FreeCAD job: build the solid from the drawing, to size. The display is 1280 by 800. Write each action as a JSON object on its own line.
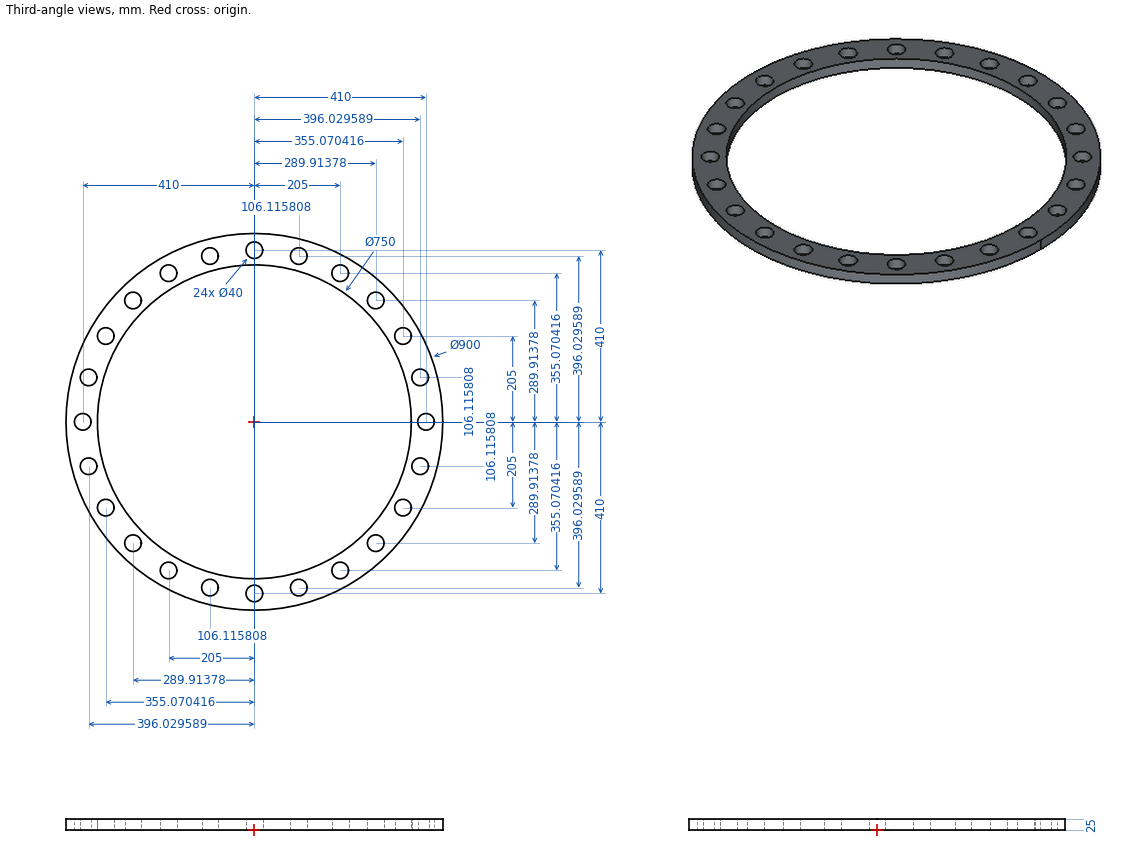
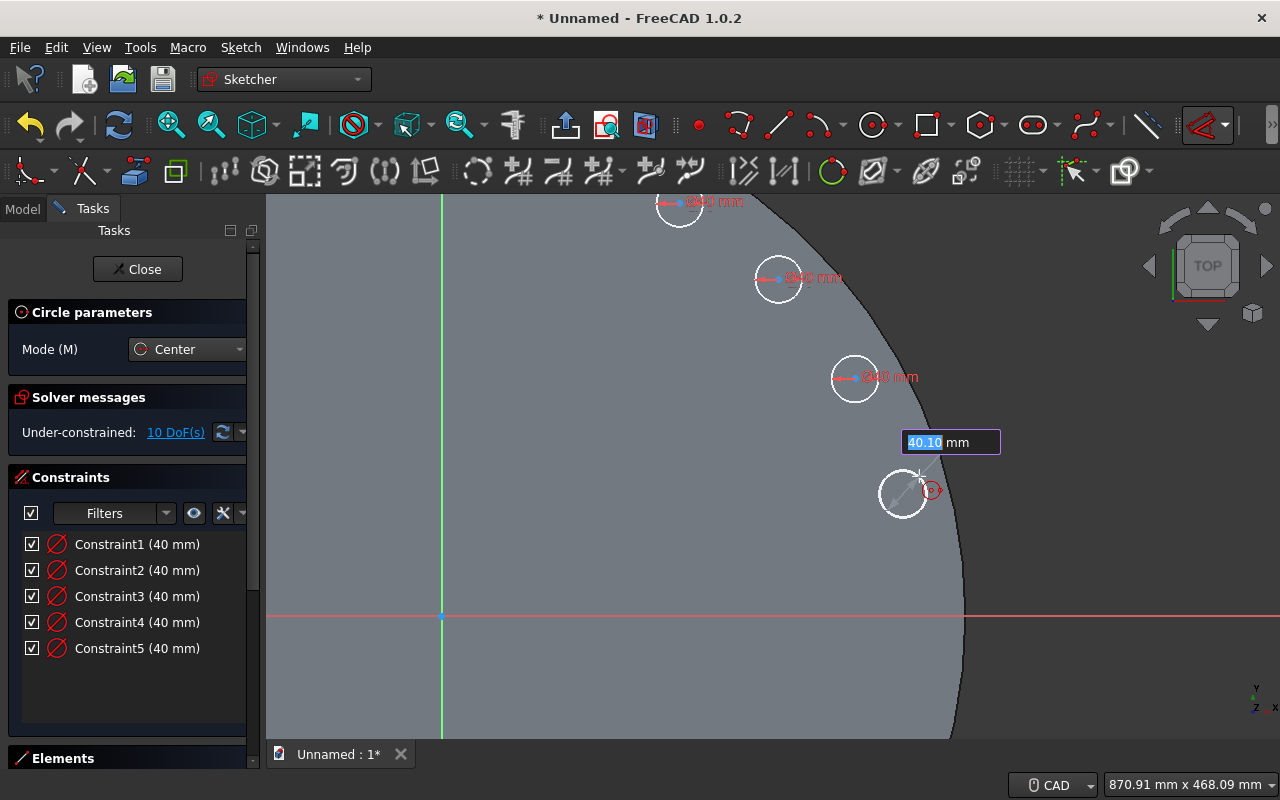
{"action": "type", "text": "40"}
{"action": "key", "text": "Return"}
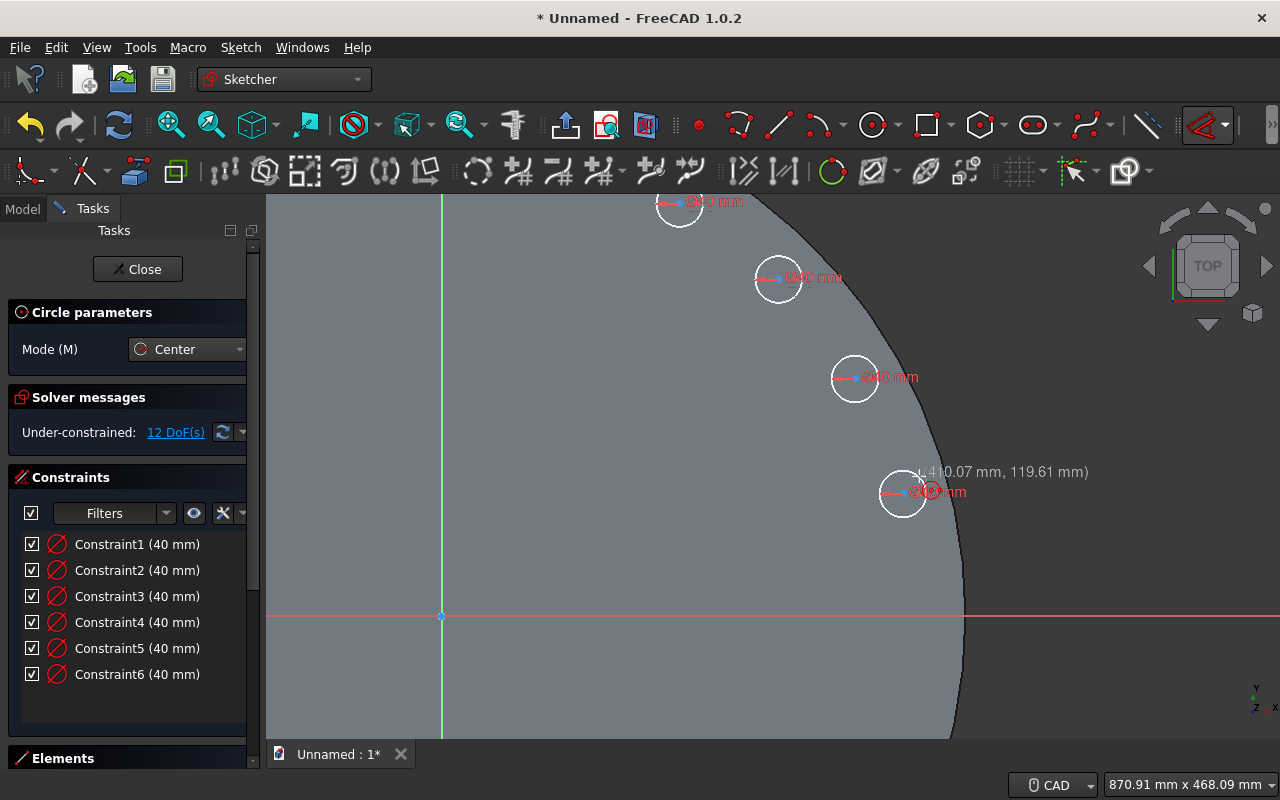
{"action": "left_click", "coordinate": [919, 616]}
{"action": "mouse_move", "coordinate": [935, 600]}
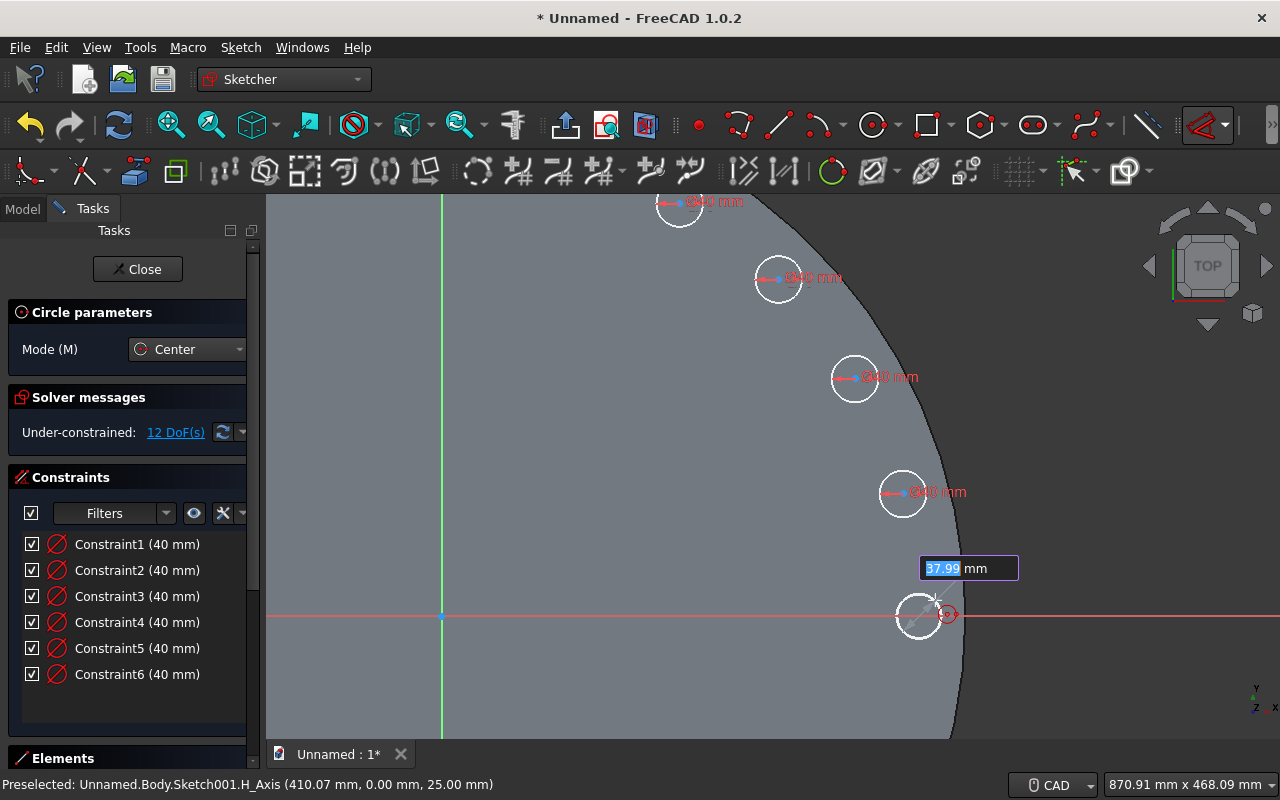
{"action": "type", "text": "40"}
{"action": "key", "text": "Return"}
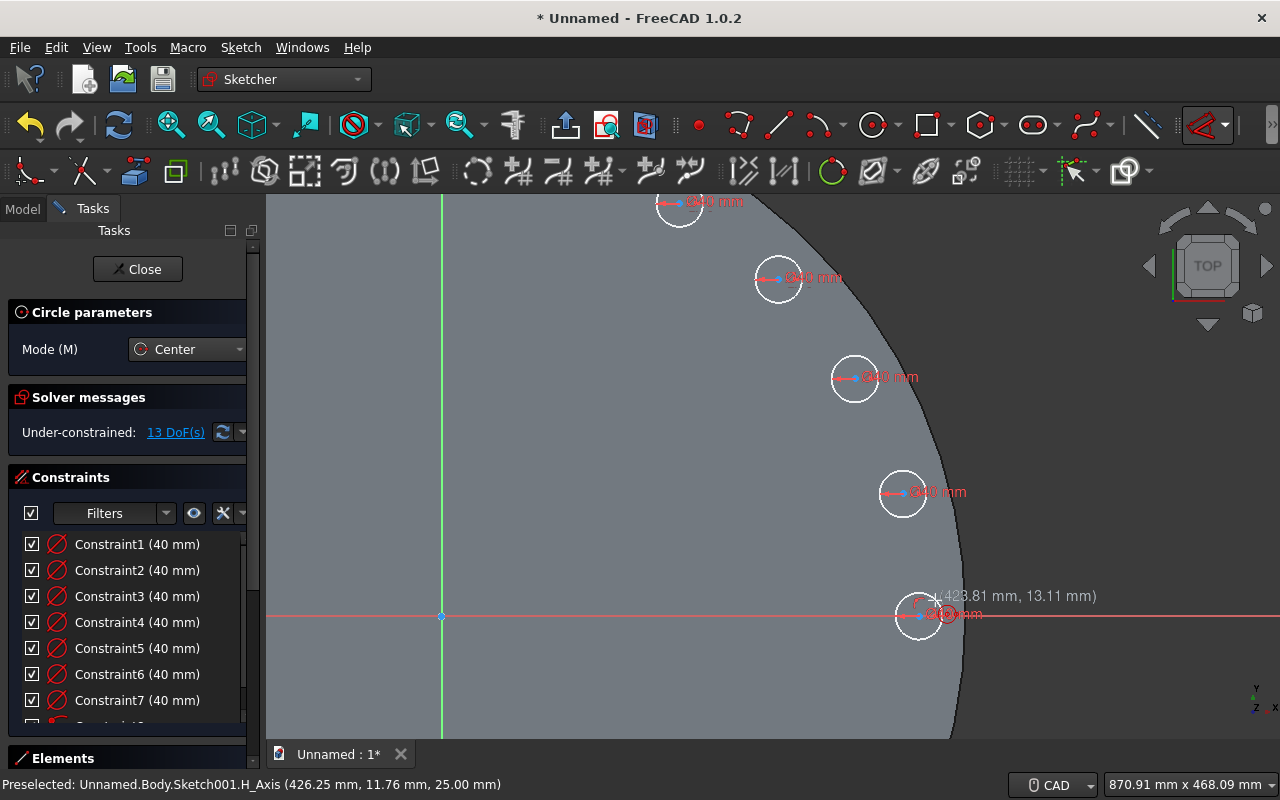
{"action": "scroll", "coordinate": [858, 379], "scroll_direction": "down", "scroll_amount": 5}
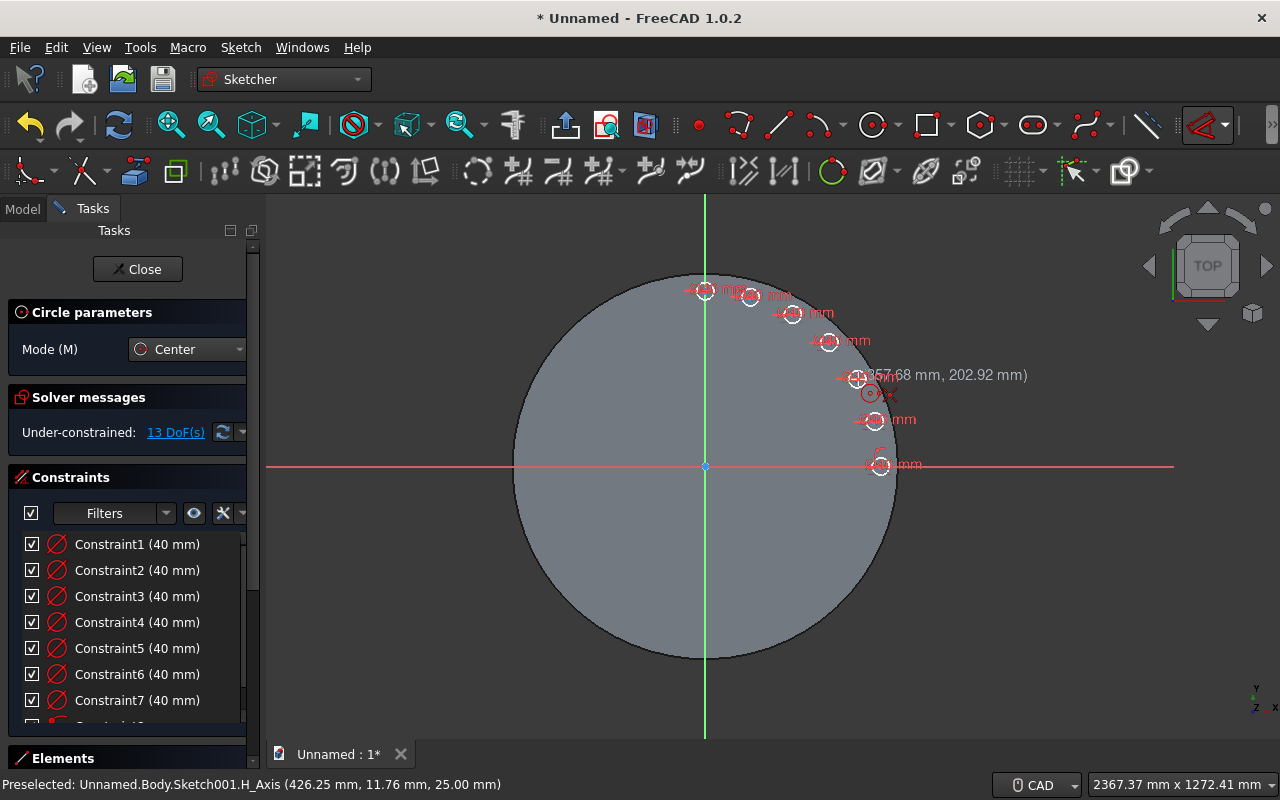
{"action": "scroll", "coordinate": [875, 512], "scroll_direction": "up", "scroll_amount": 5}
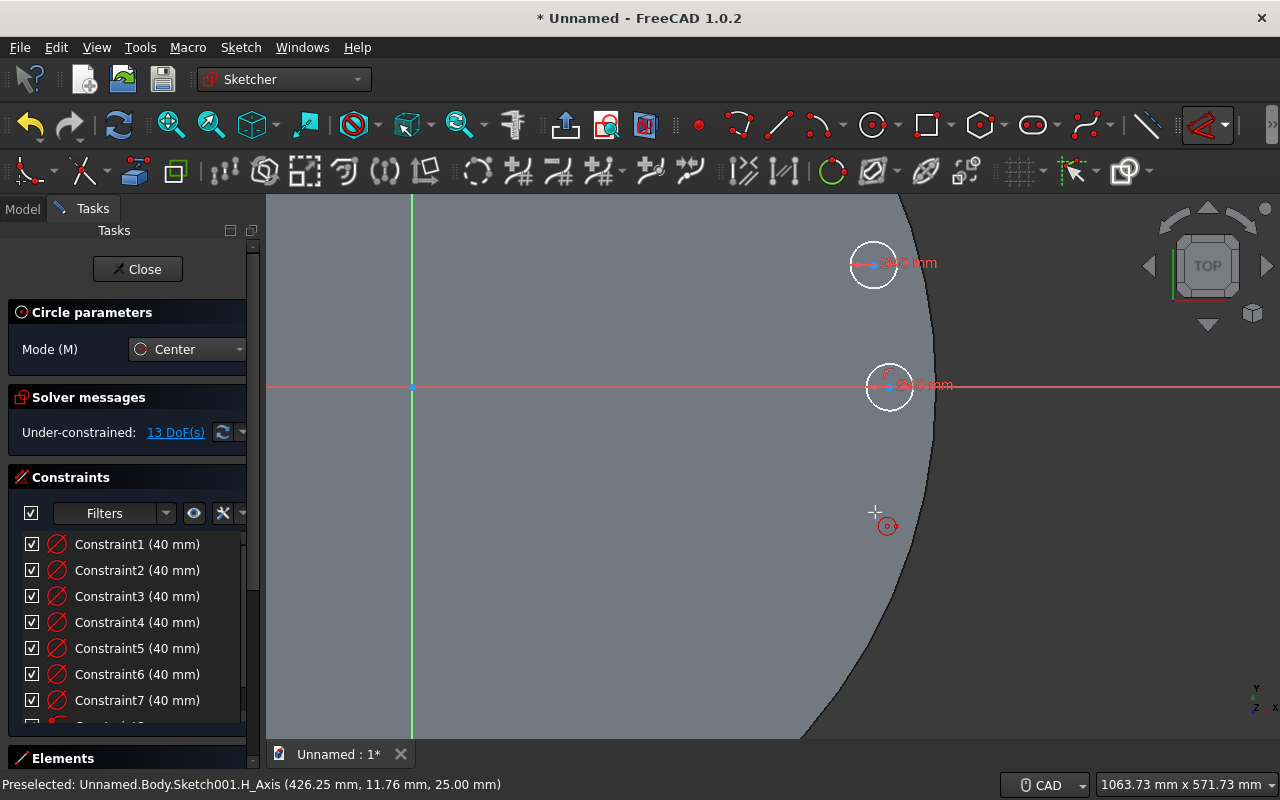
{"action": "left_click", "coordinate": [873, 511]}
{"action": "mouse_move", "coordinate": [890, 494]}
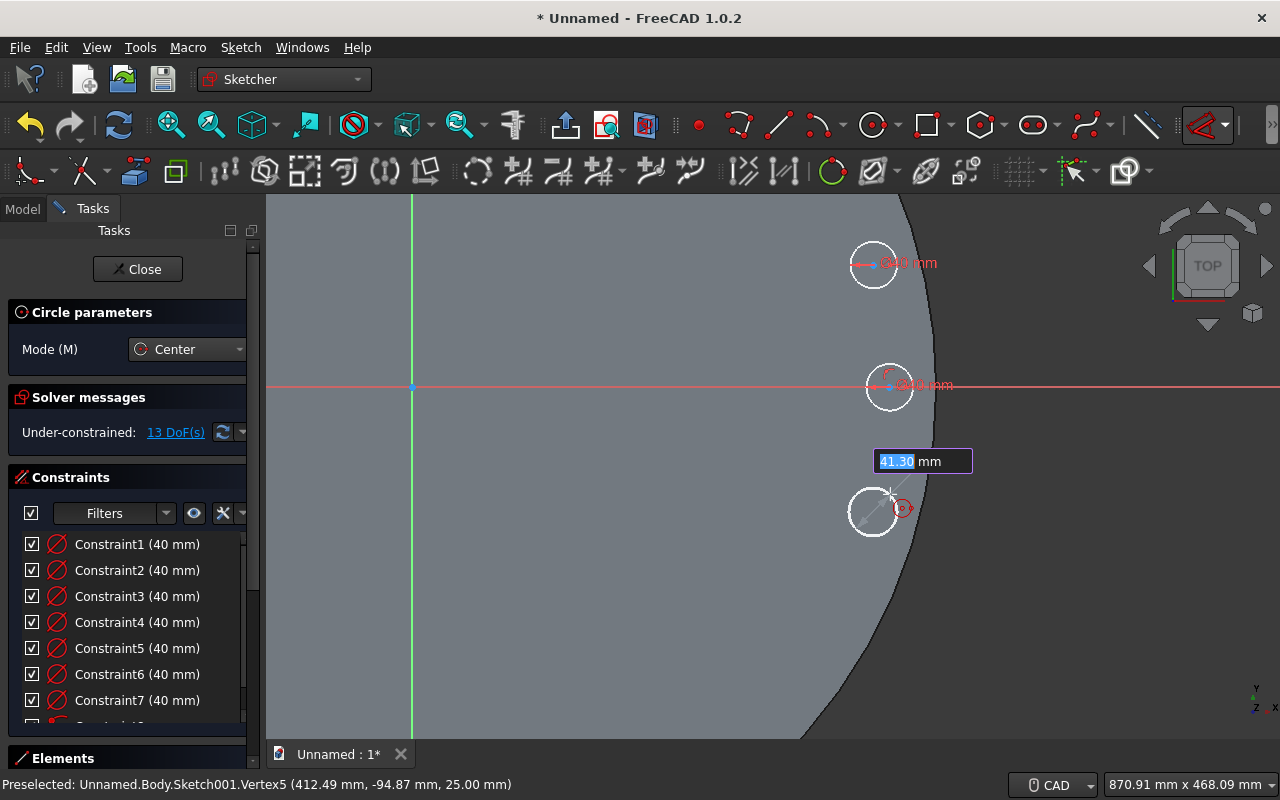
{"action": "type", "text": "40"}
{"action": "key", "text": "Return"}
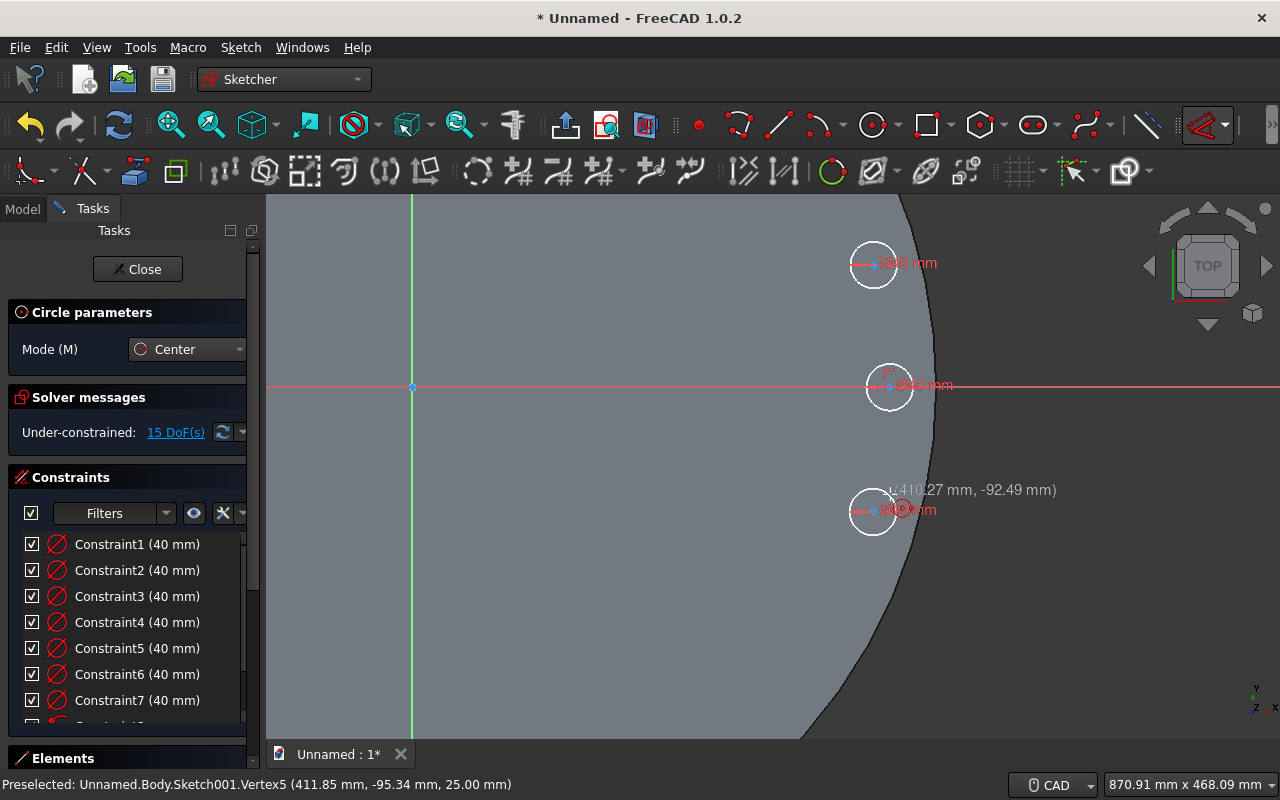
{"action": "left_click", "coordinate": [826, 626]}
{"action": "mouse_move", "coordinate": [842, 610]}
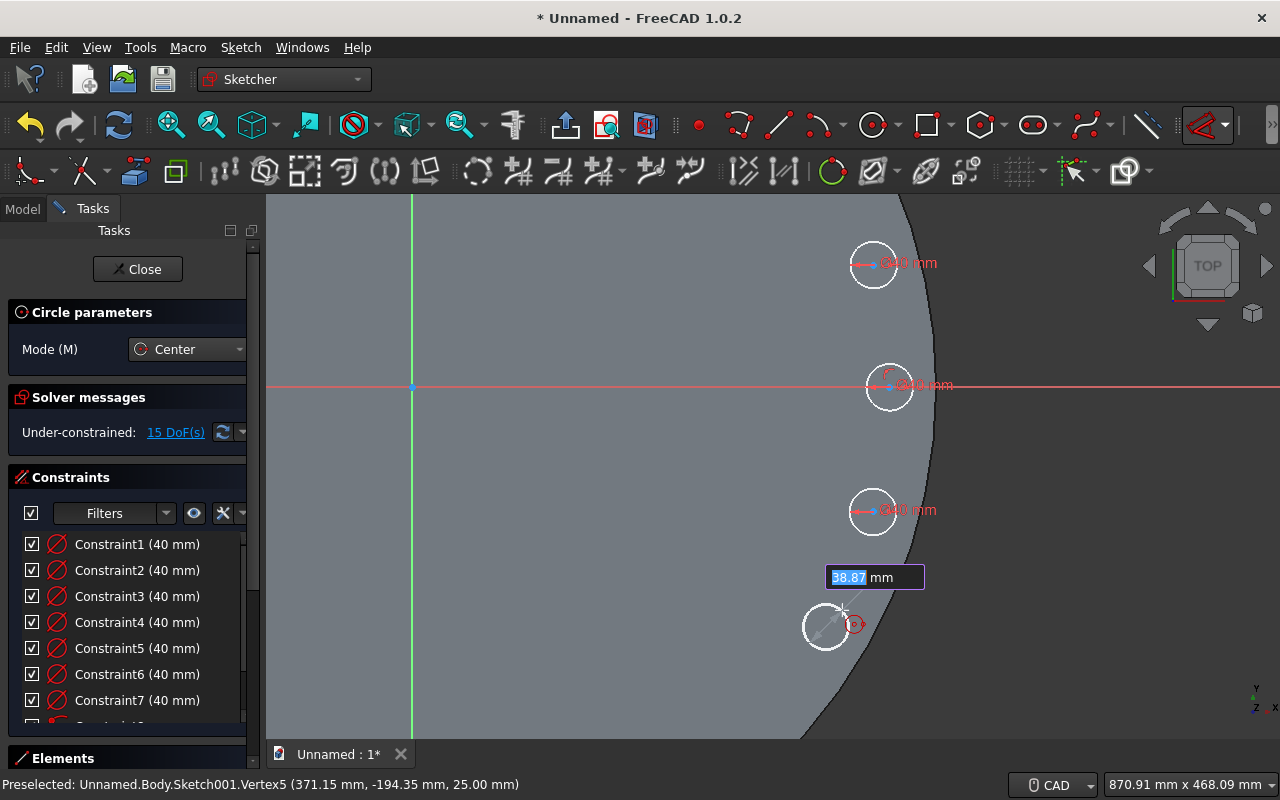
{"action": "type", "text": "40"}
{"action": "key", "text": "Return"}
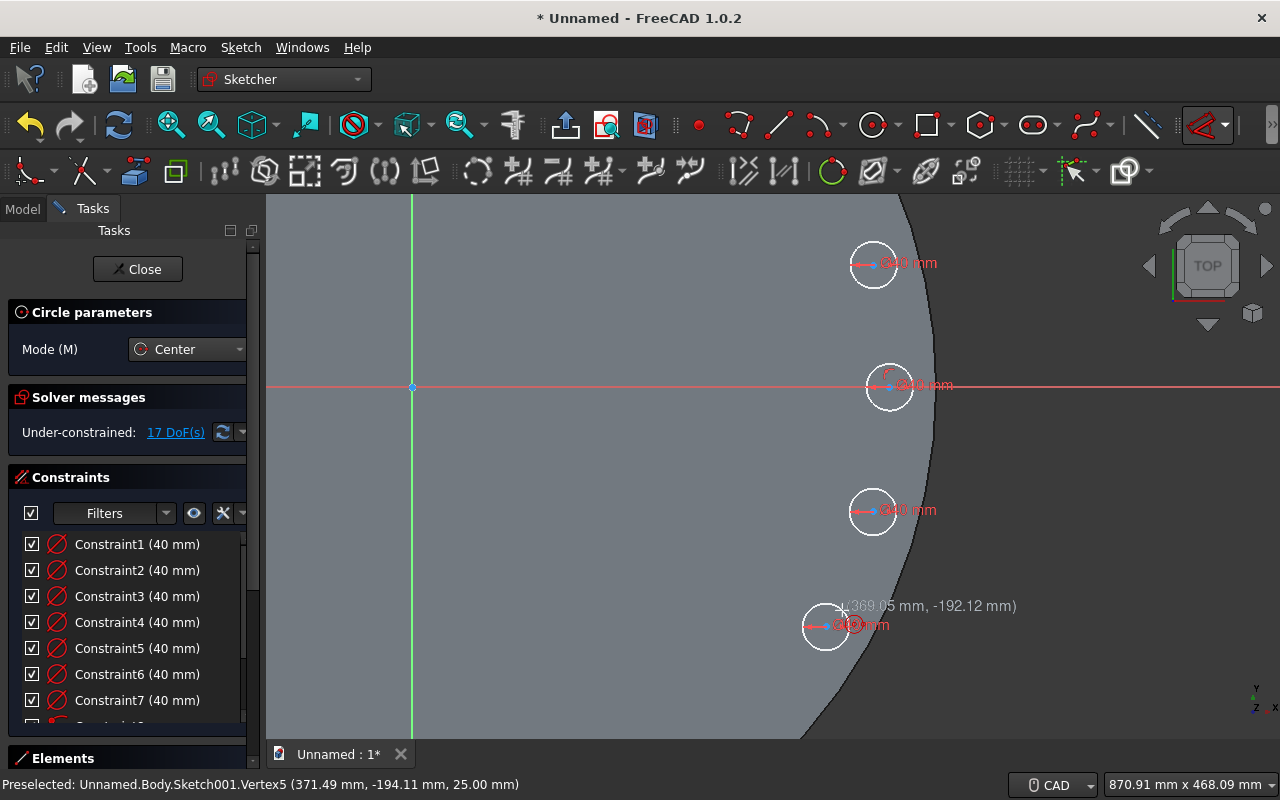
{"action": "scroll", "coordinate": [875, 513], "scroll_direction": "down", "scroll_amount": 5}